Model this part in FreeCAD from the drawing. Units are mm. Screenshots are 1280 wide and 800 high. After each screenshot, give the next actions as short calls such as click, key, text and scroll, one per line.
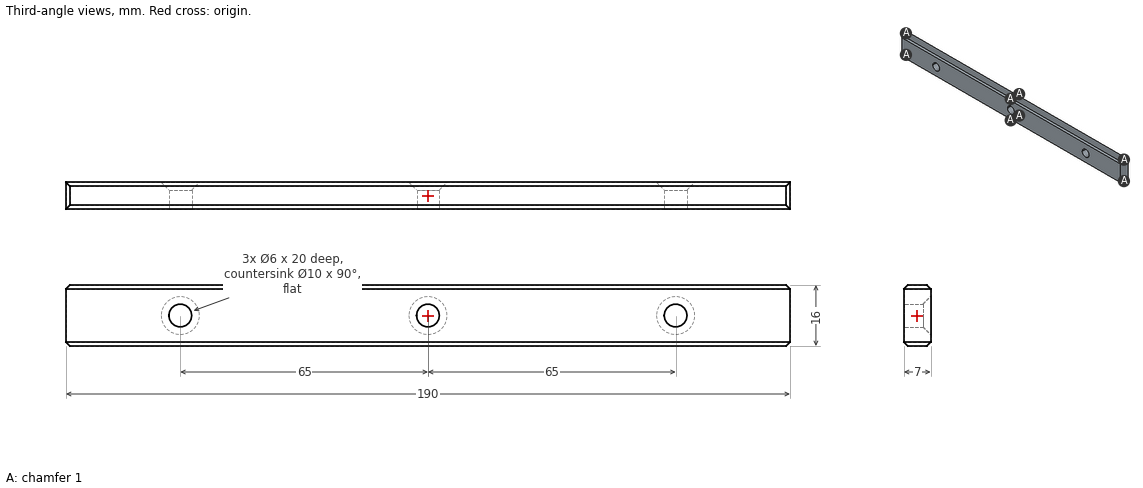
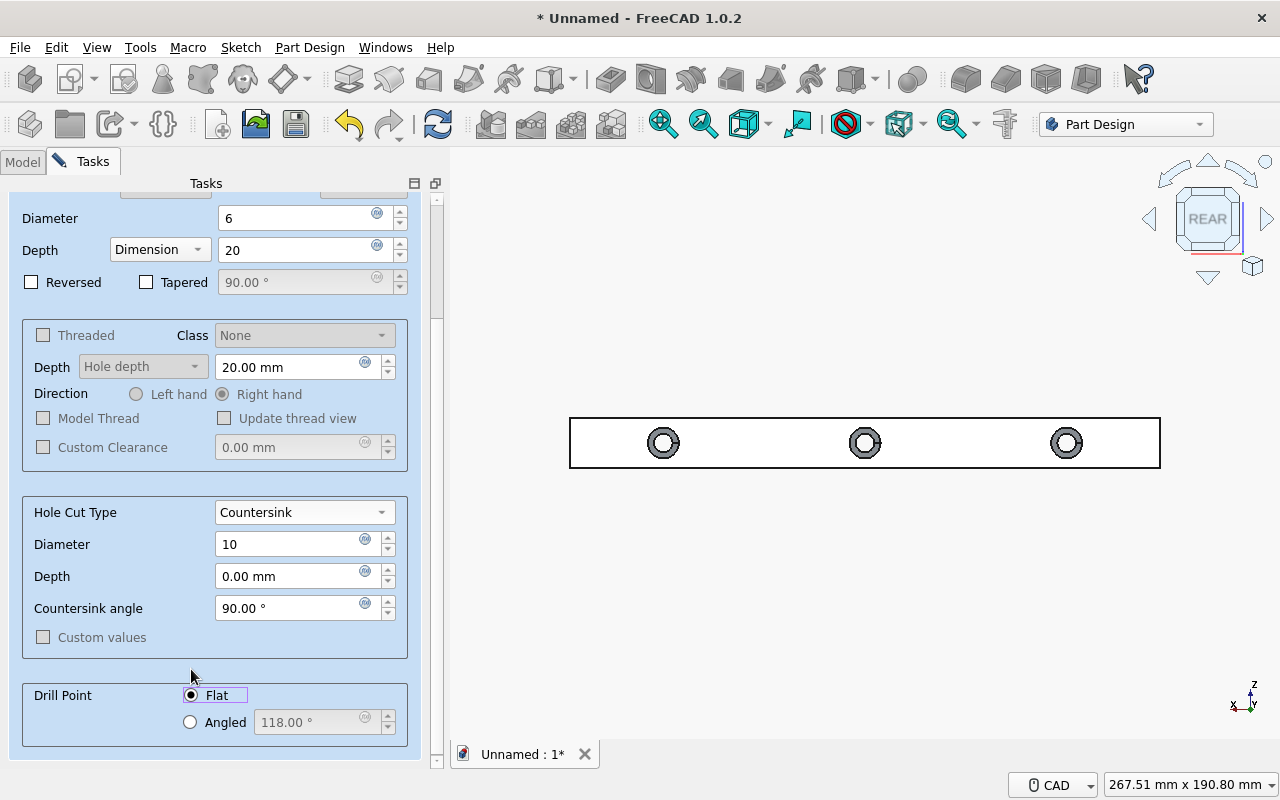
scroll(437, 480, up, 4)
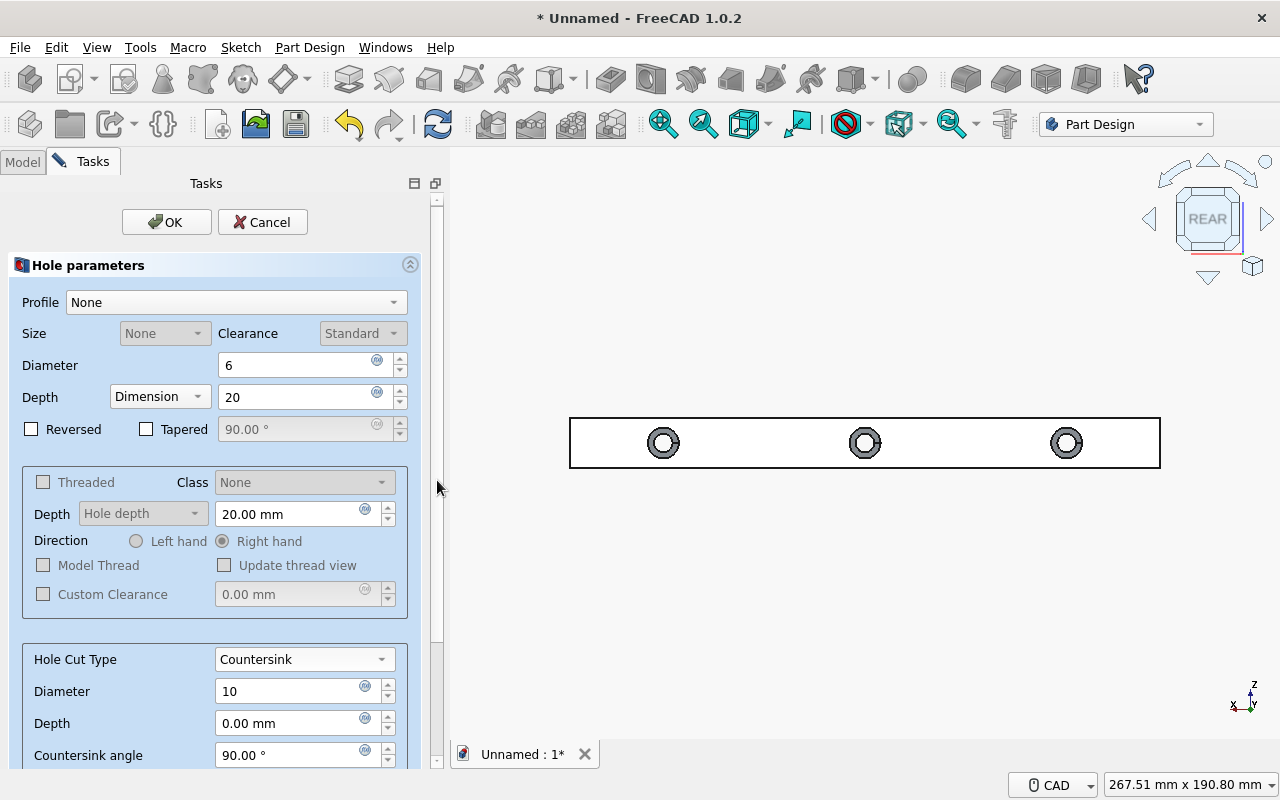
click(167, 222)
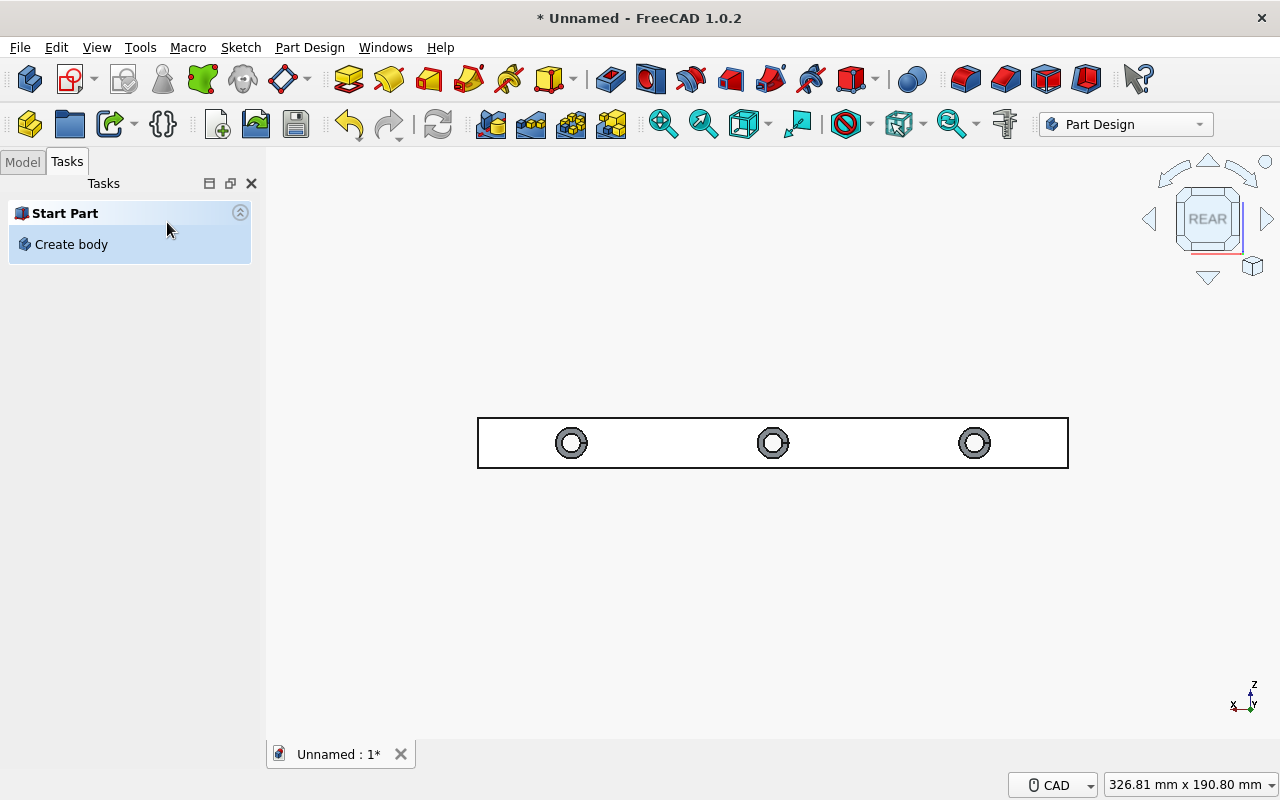
key(0)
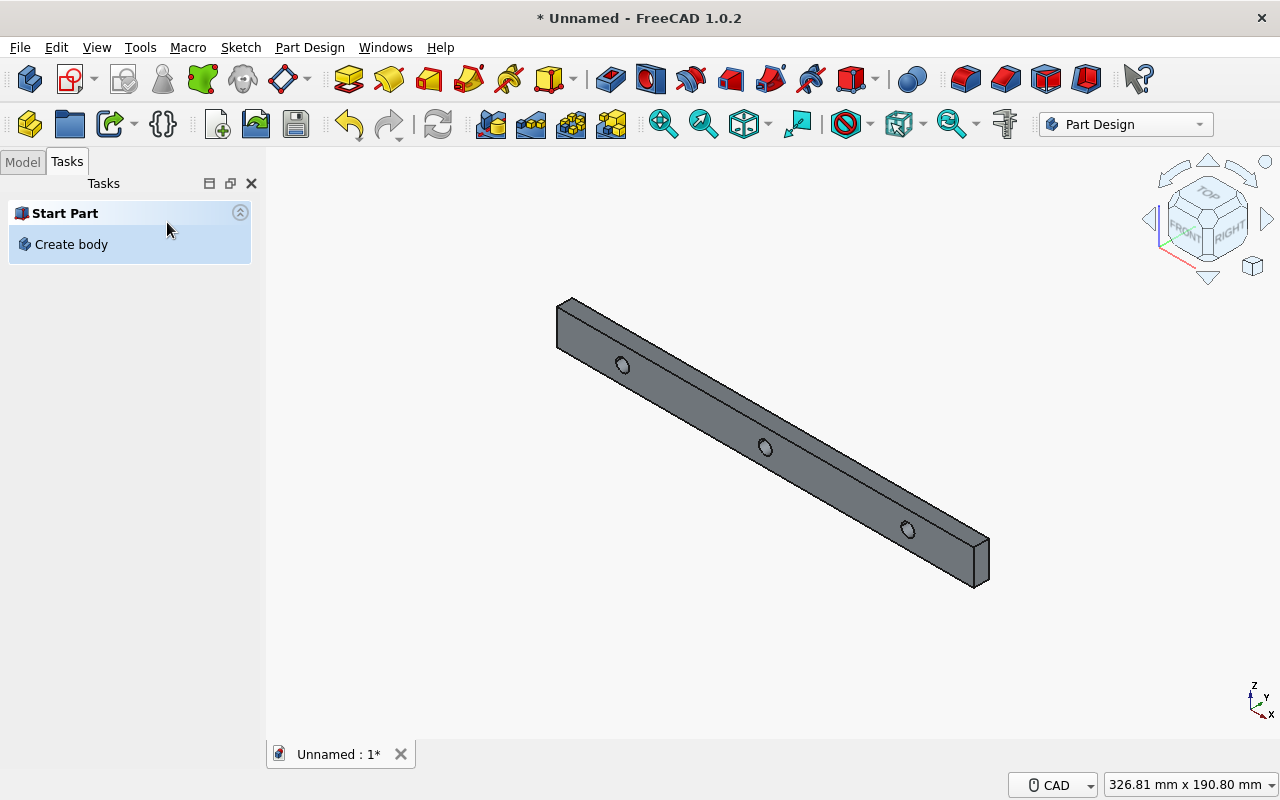
click(954, 524)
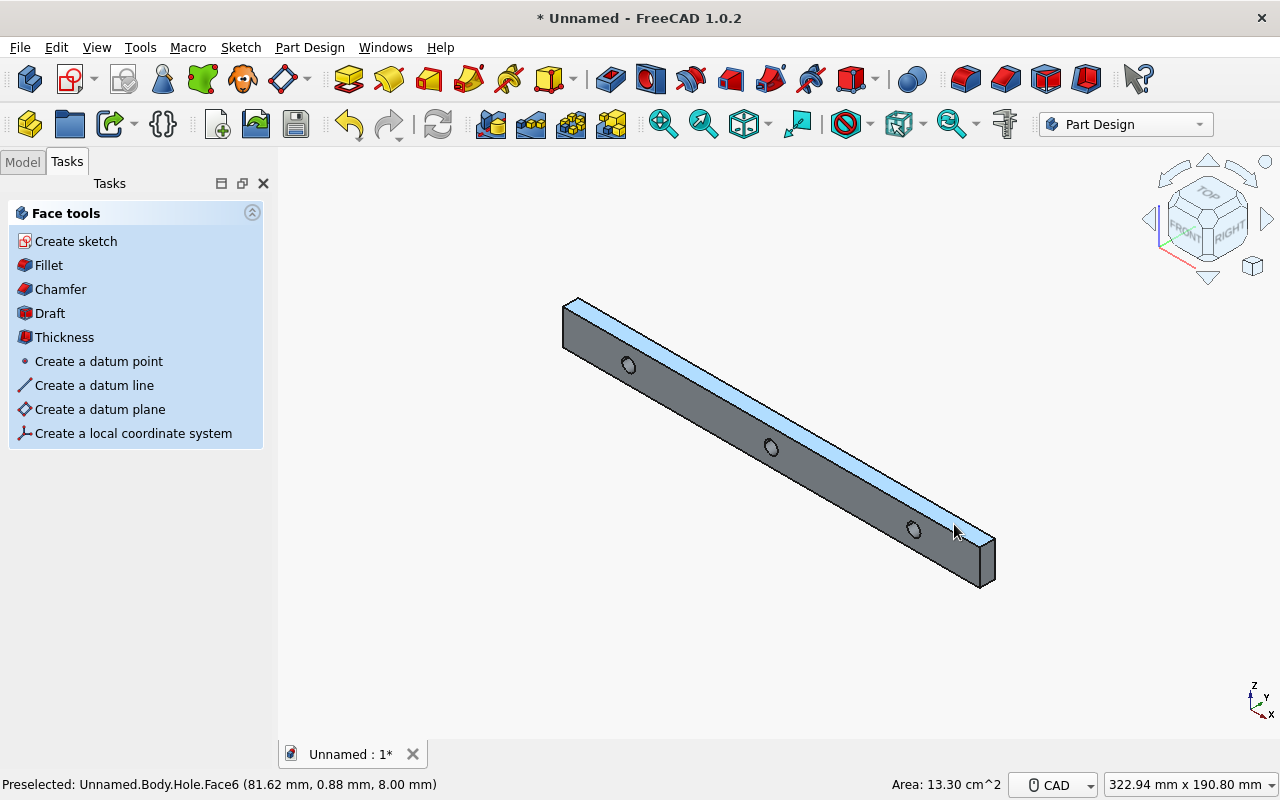
key(2)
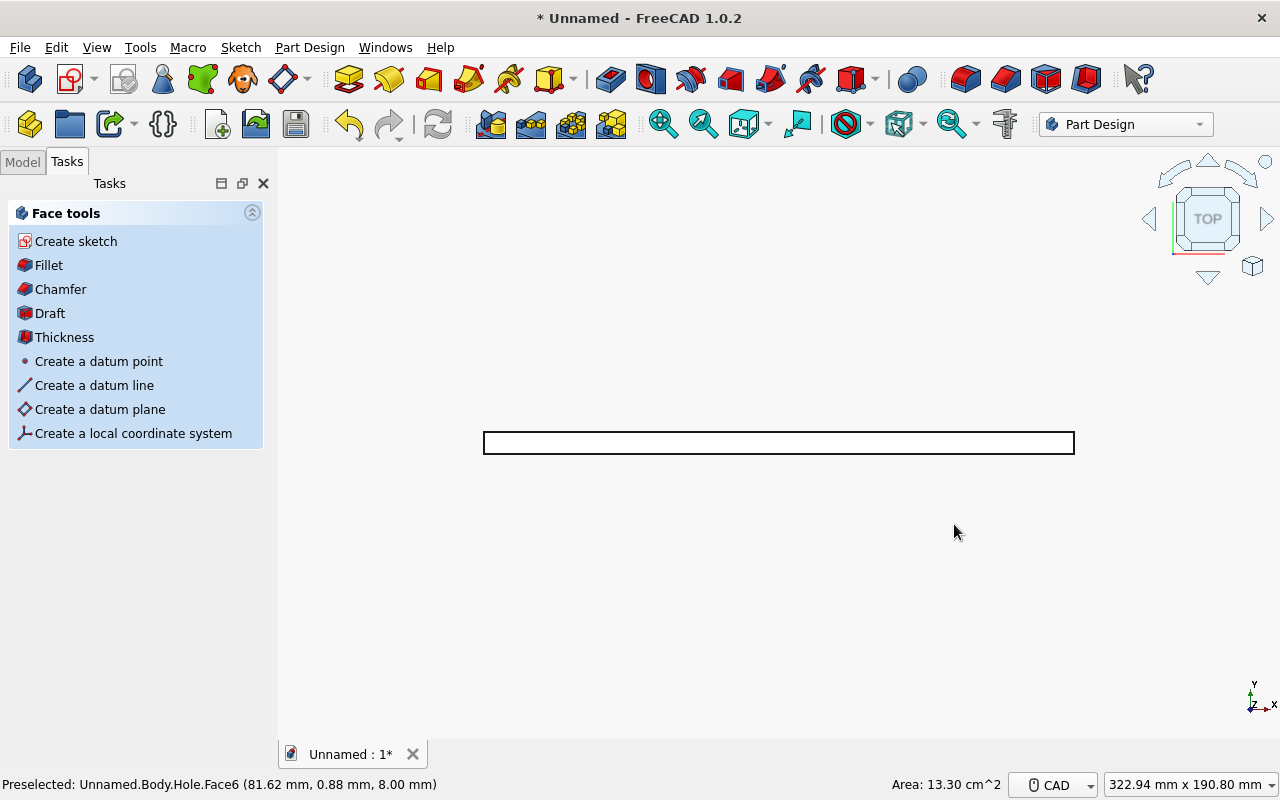
key(1)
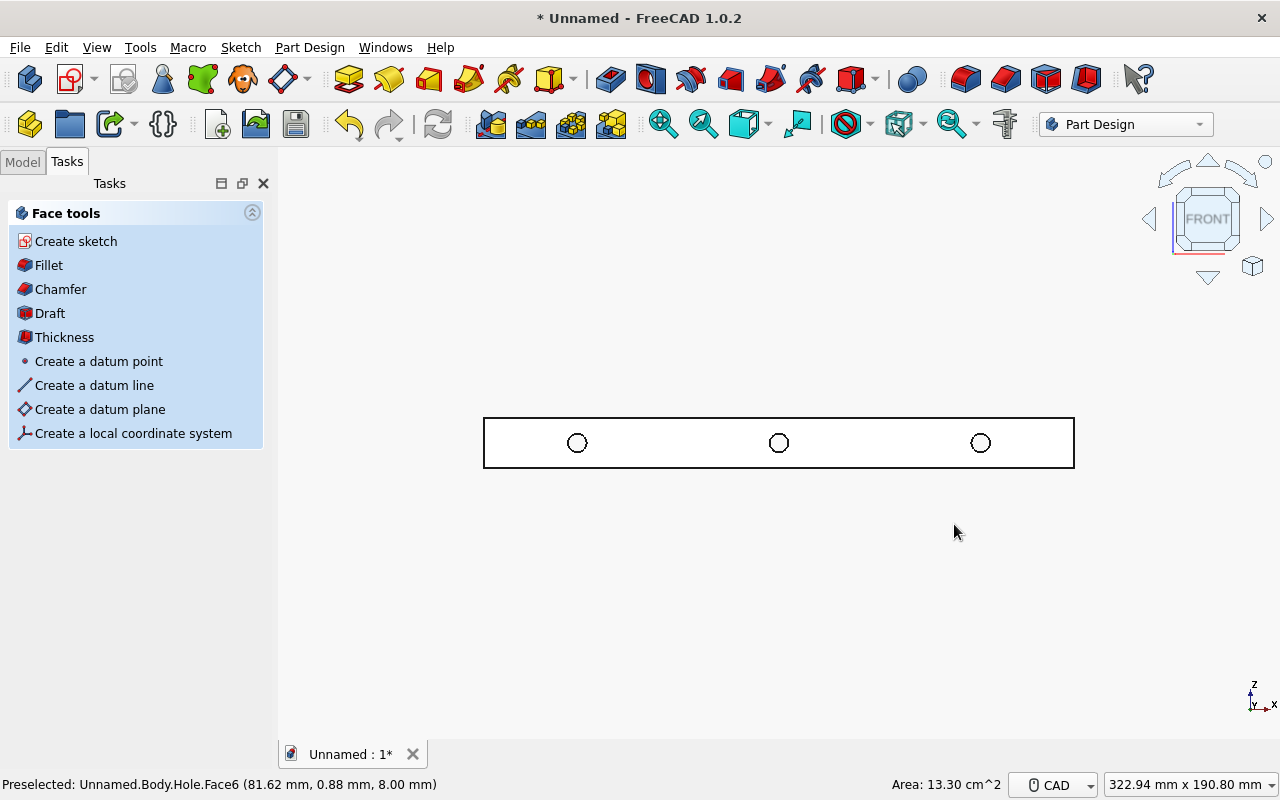
key(3)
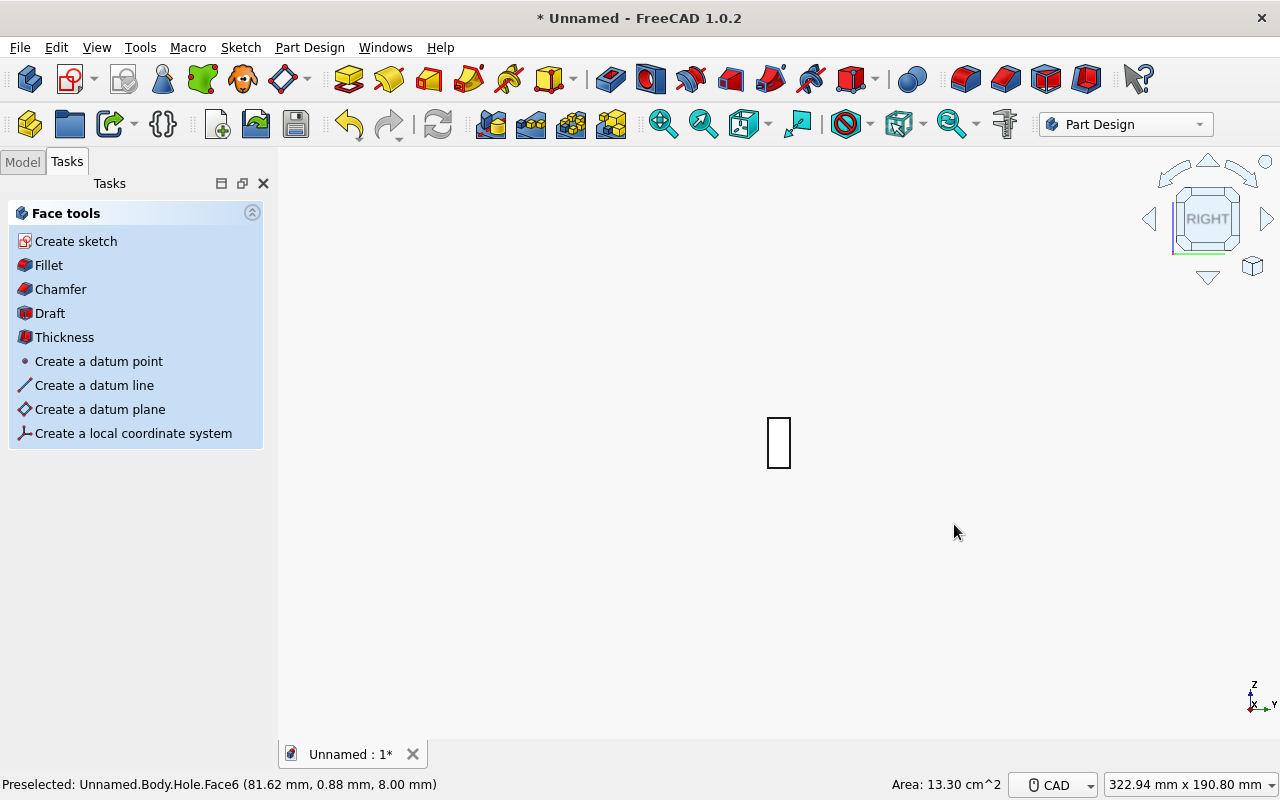
click(664, 124)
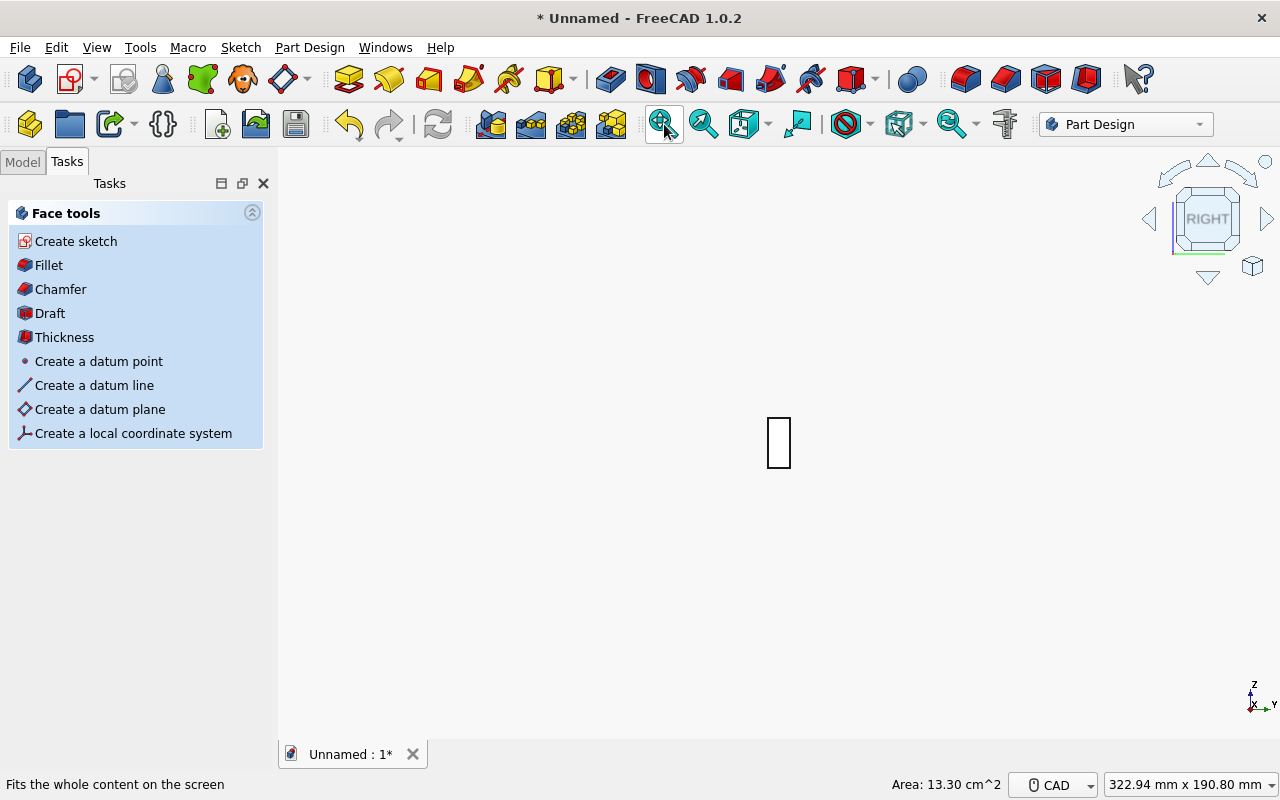
key(5)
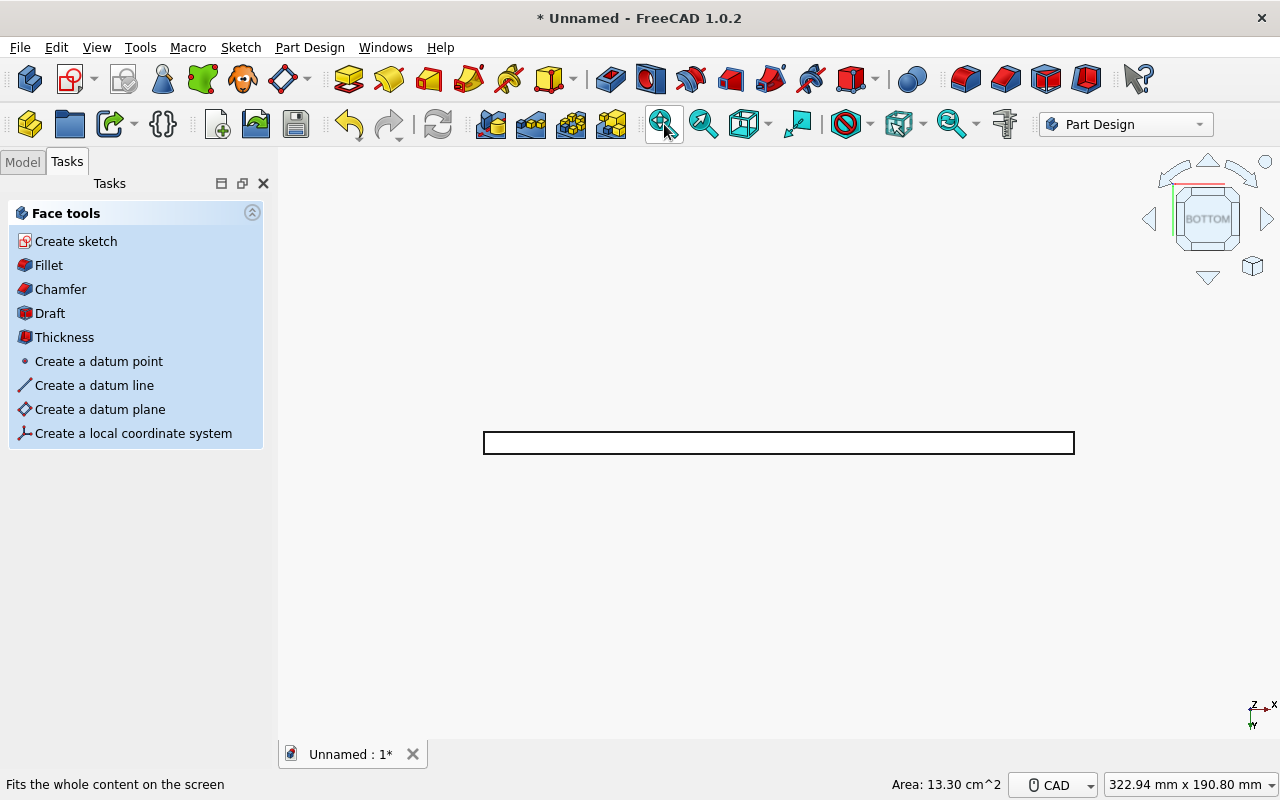
click(1032, 442, ctrl)